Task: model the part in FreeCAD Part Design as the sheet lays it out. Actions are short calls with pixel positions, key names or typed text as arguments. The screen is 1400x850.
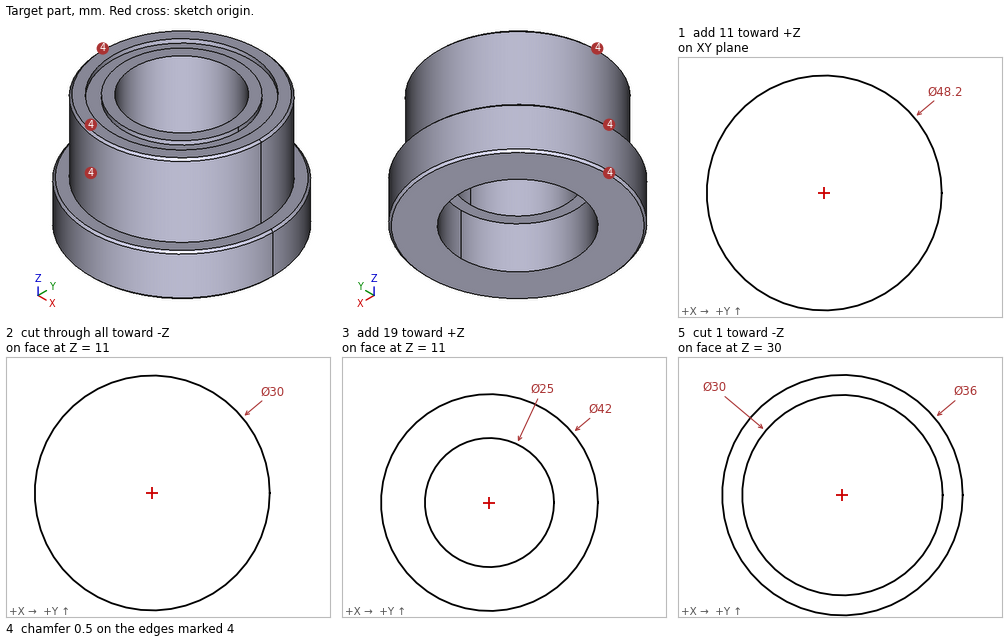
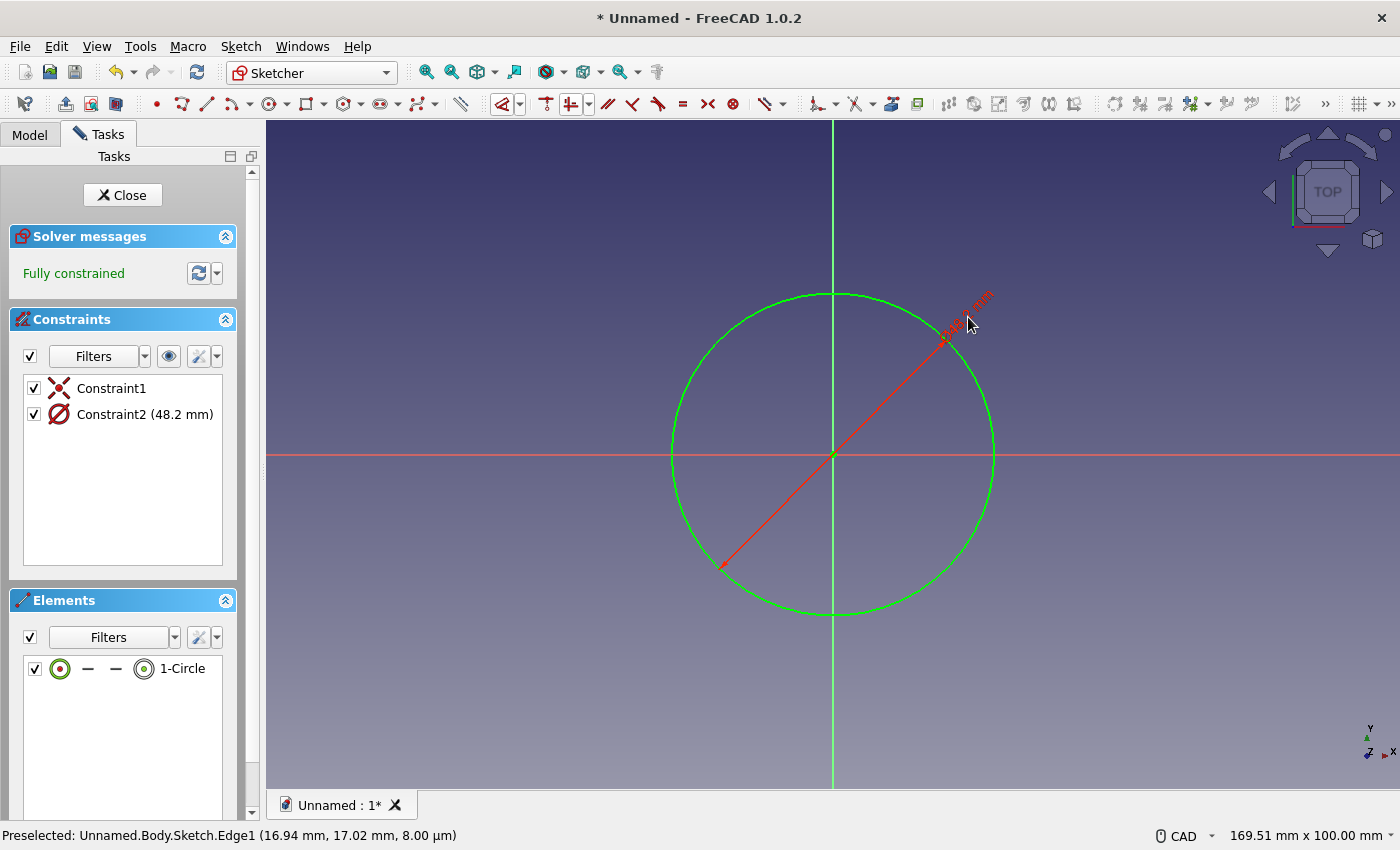
click(123, 195)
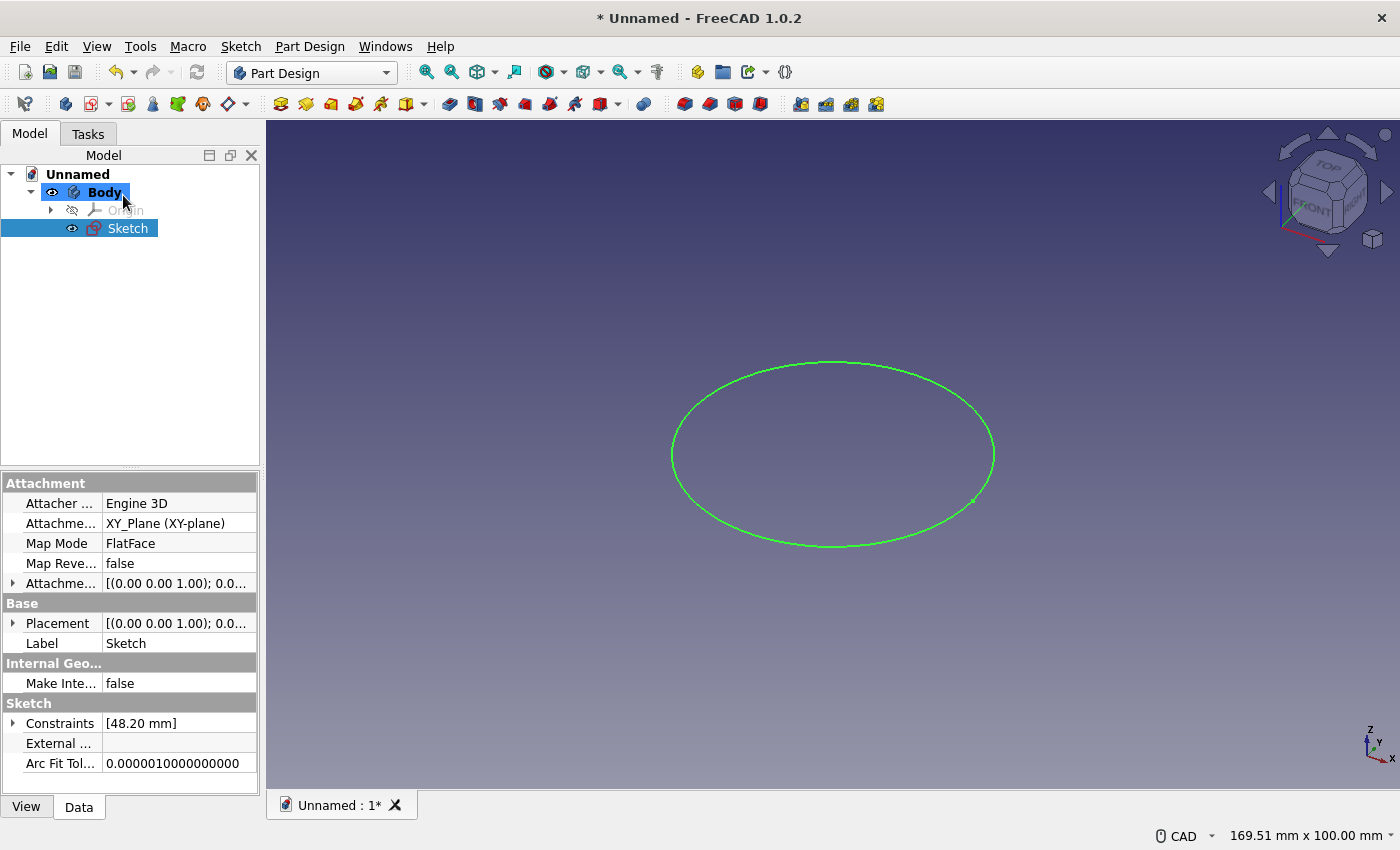
click(281, 104)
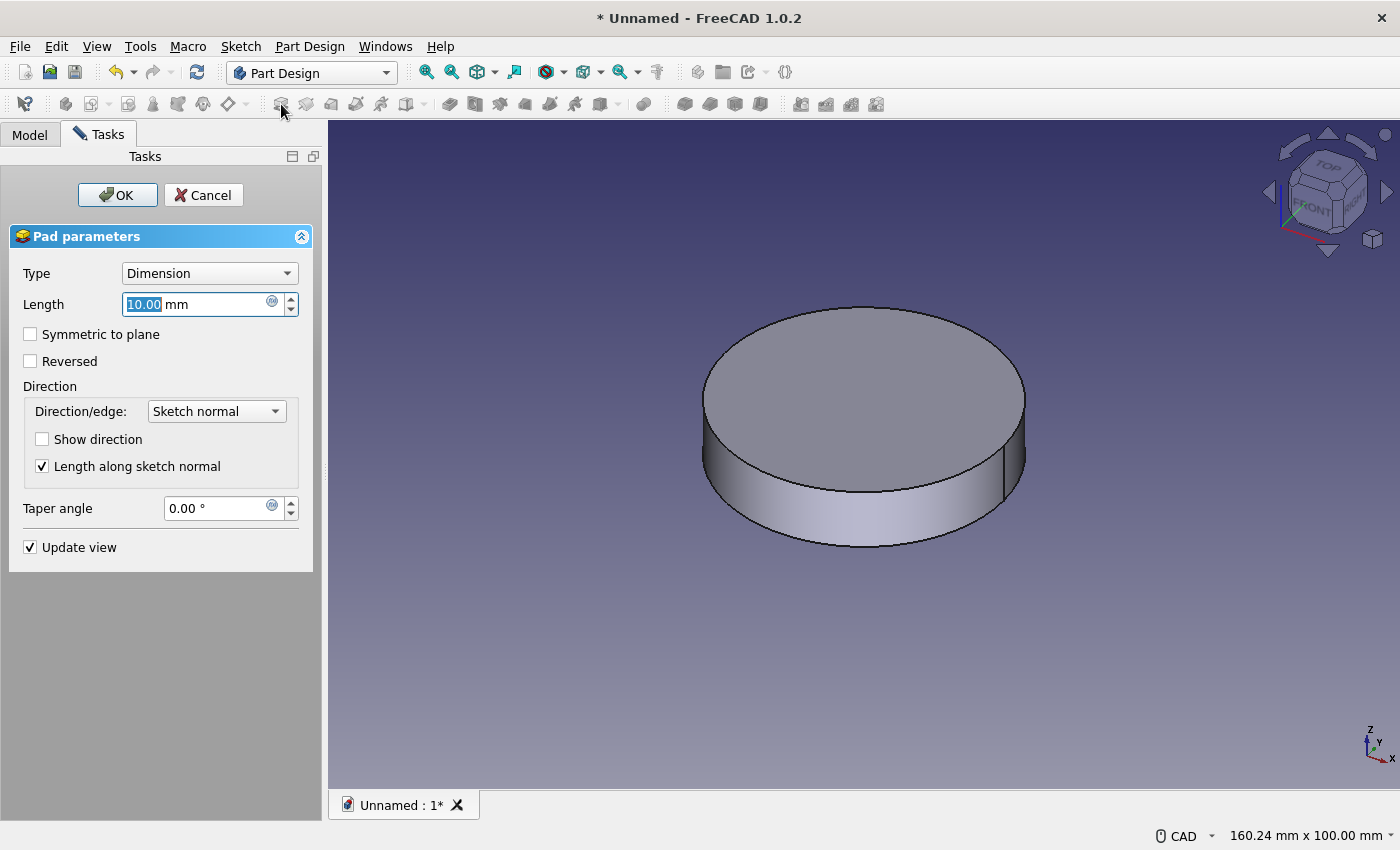
text(11)
key(Tab)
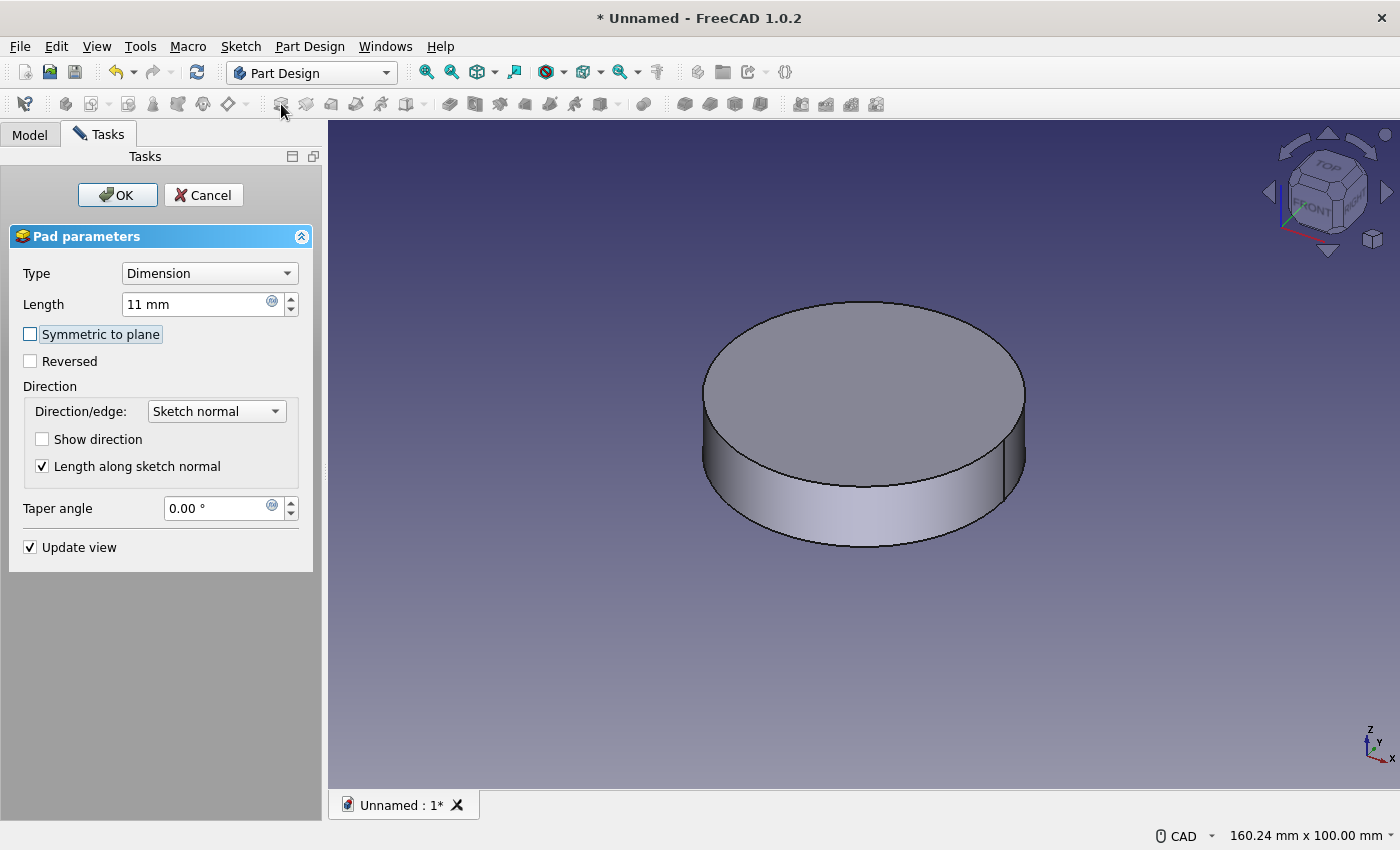
click(118, 195)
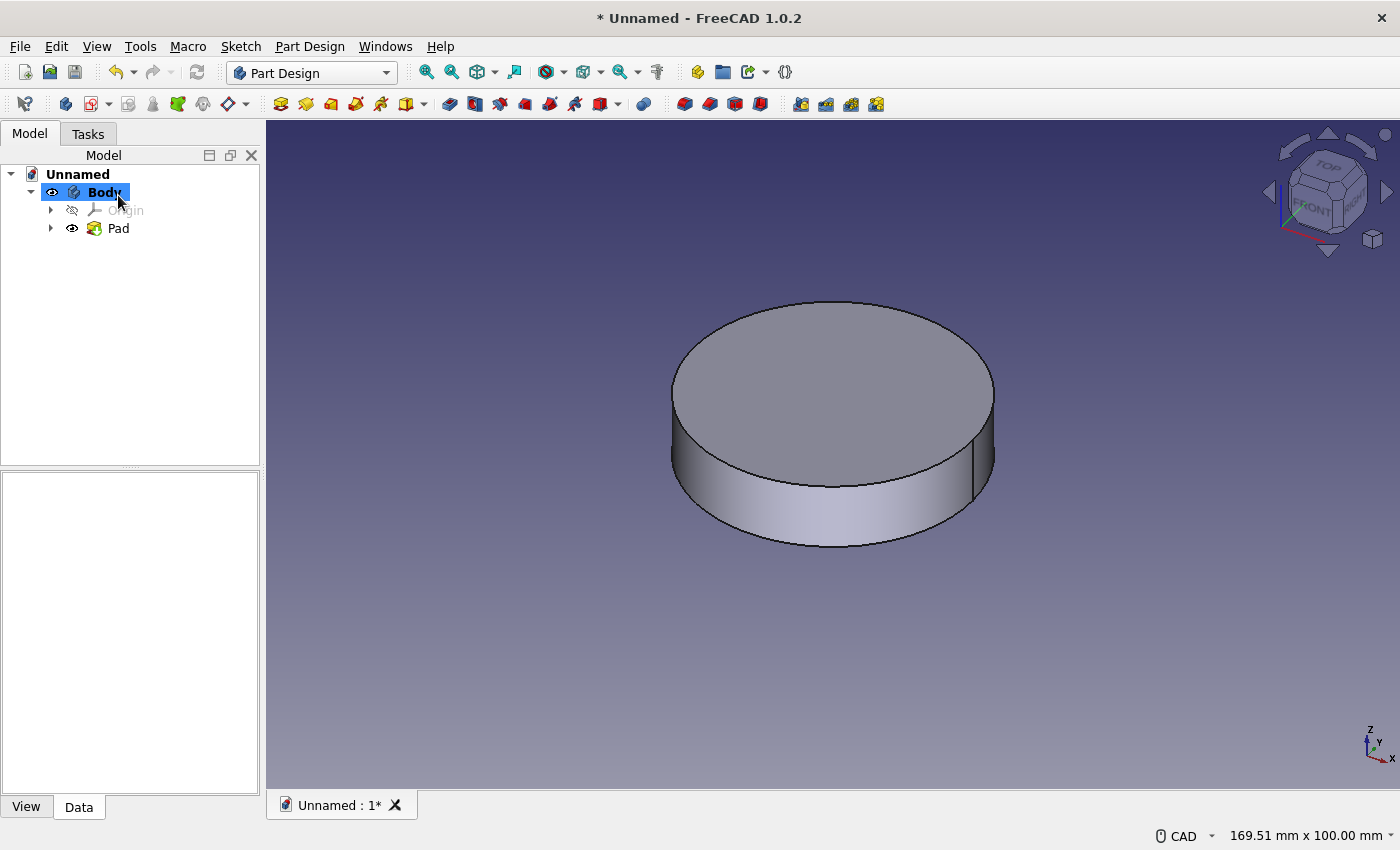
click(833, 393)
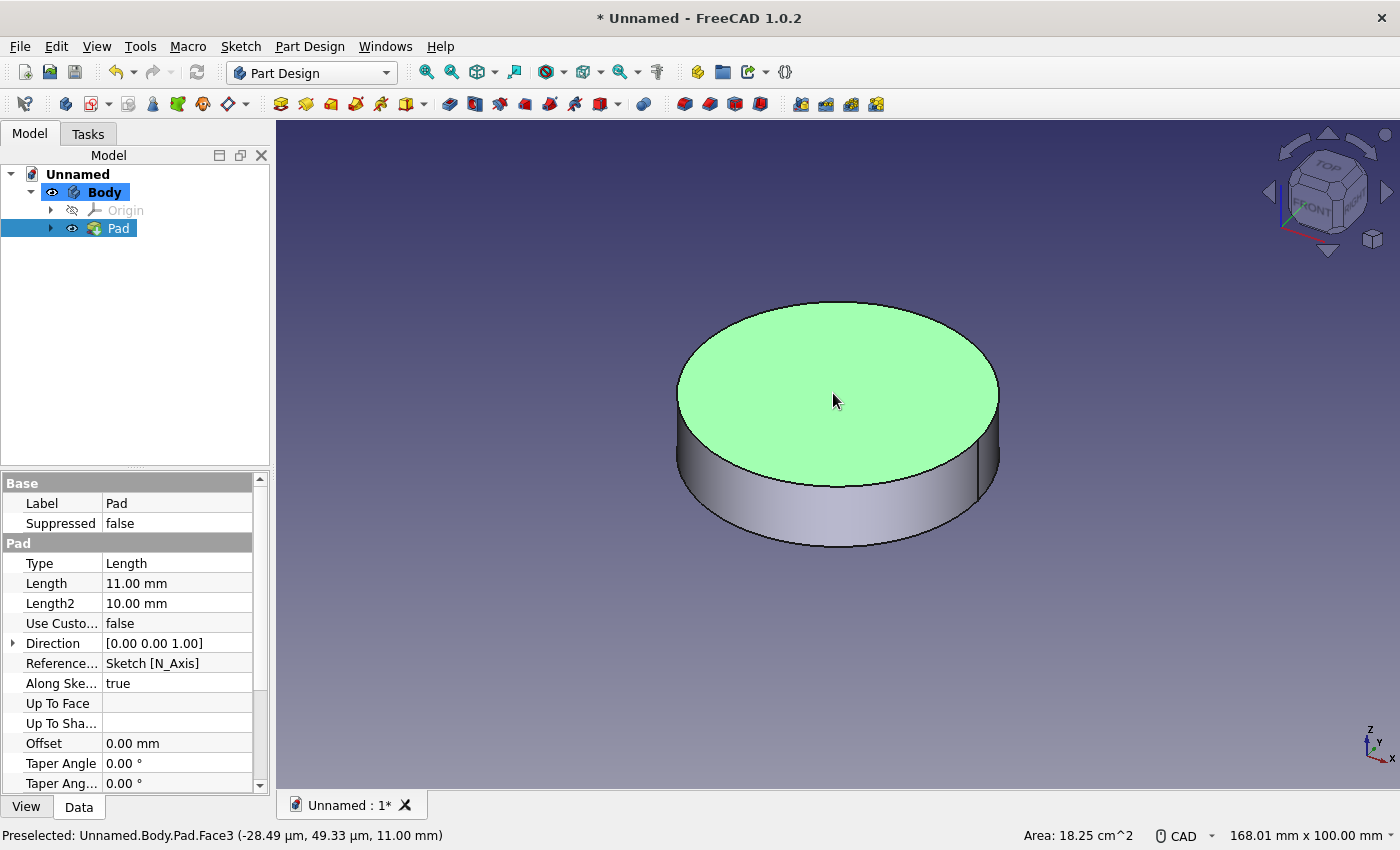
click(90, 104)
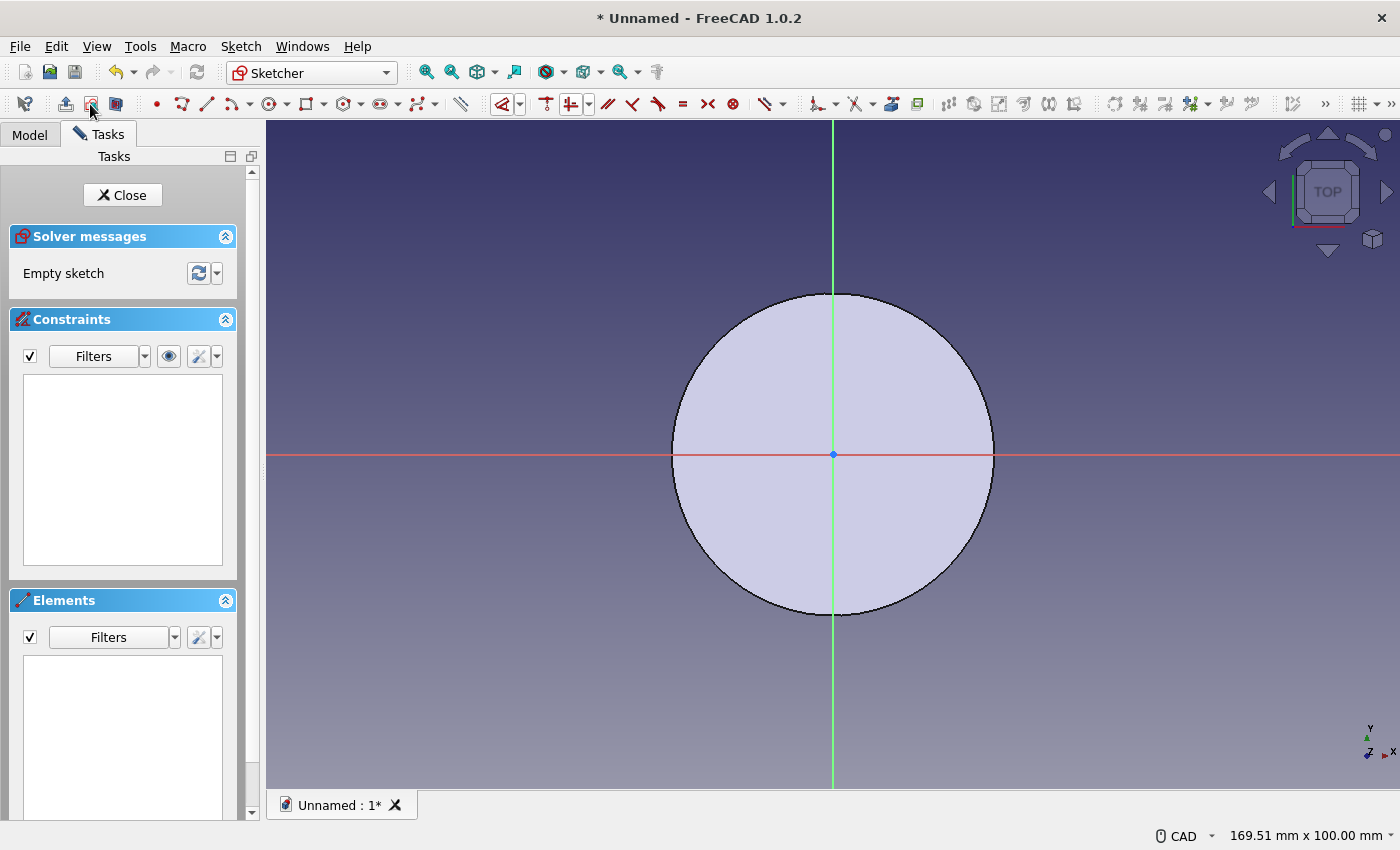
scroll(889, 455, up, 4)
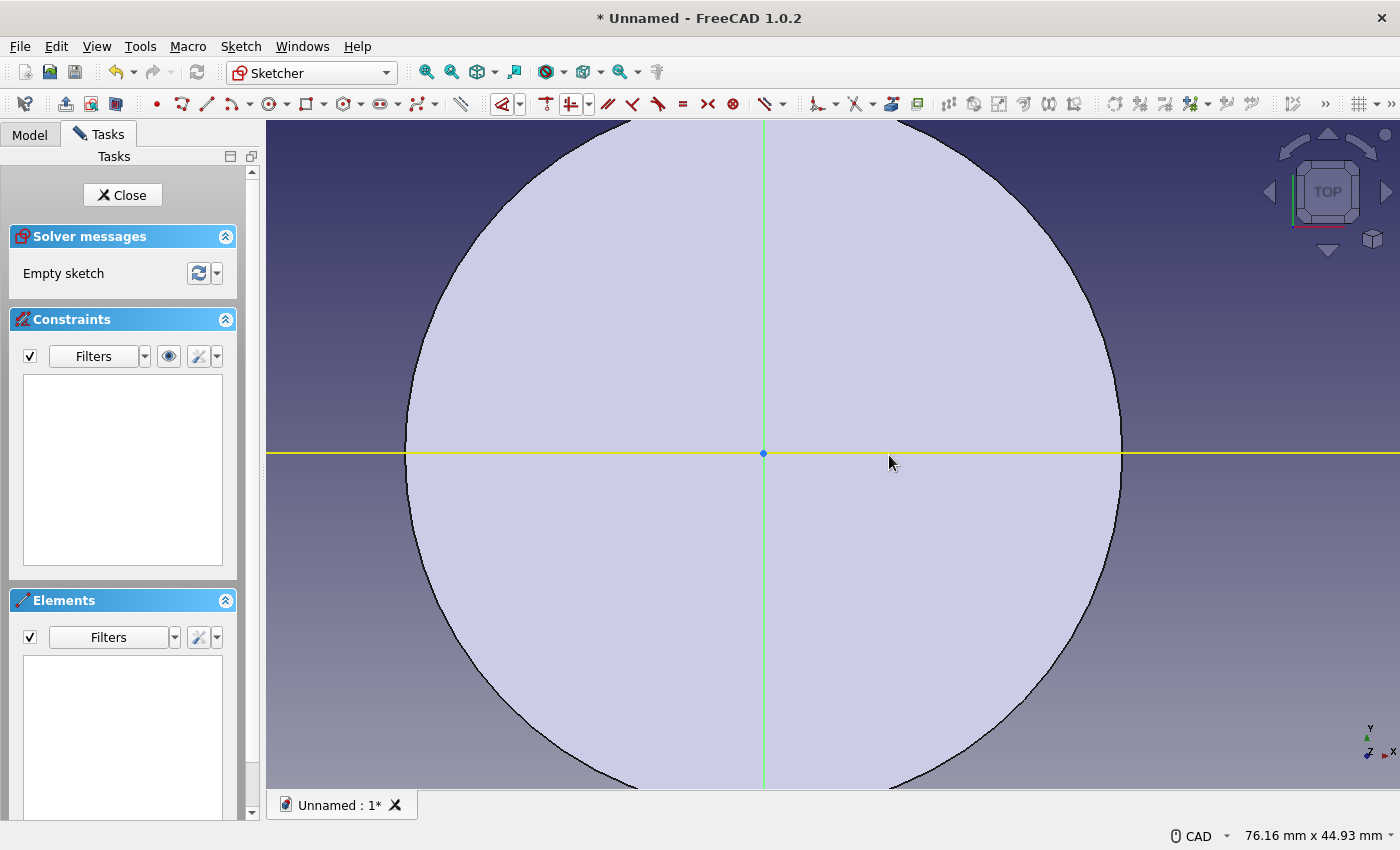
click(268, 104)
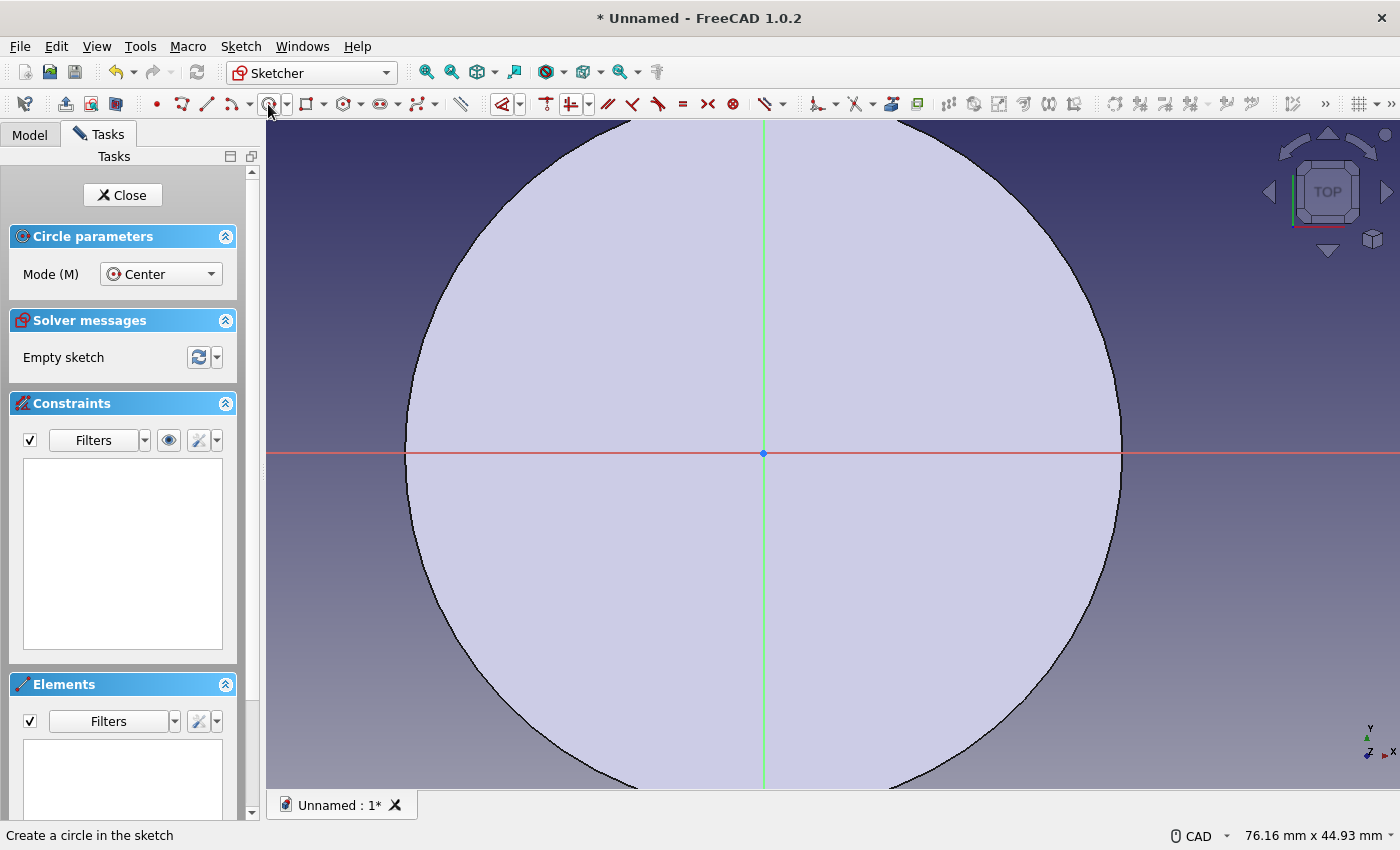
click(764, 453)
click(922, 295)
key(Escape)